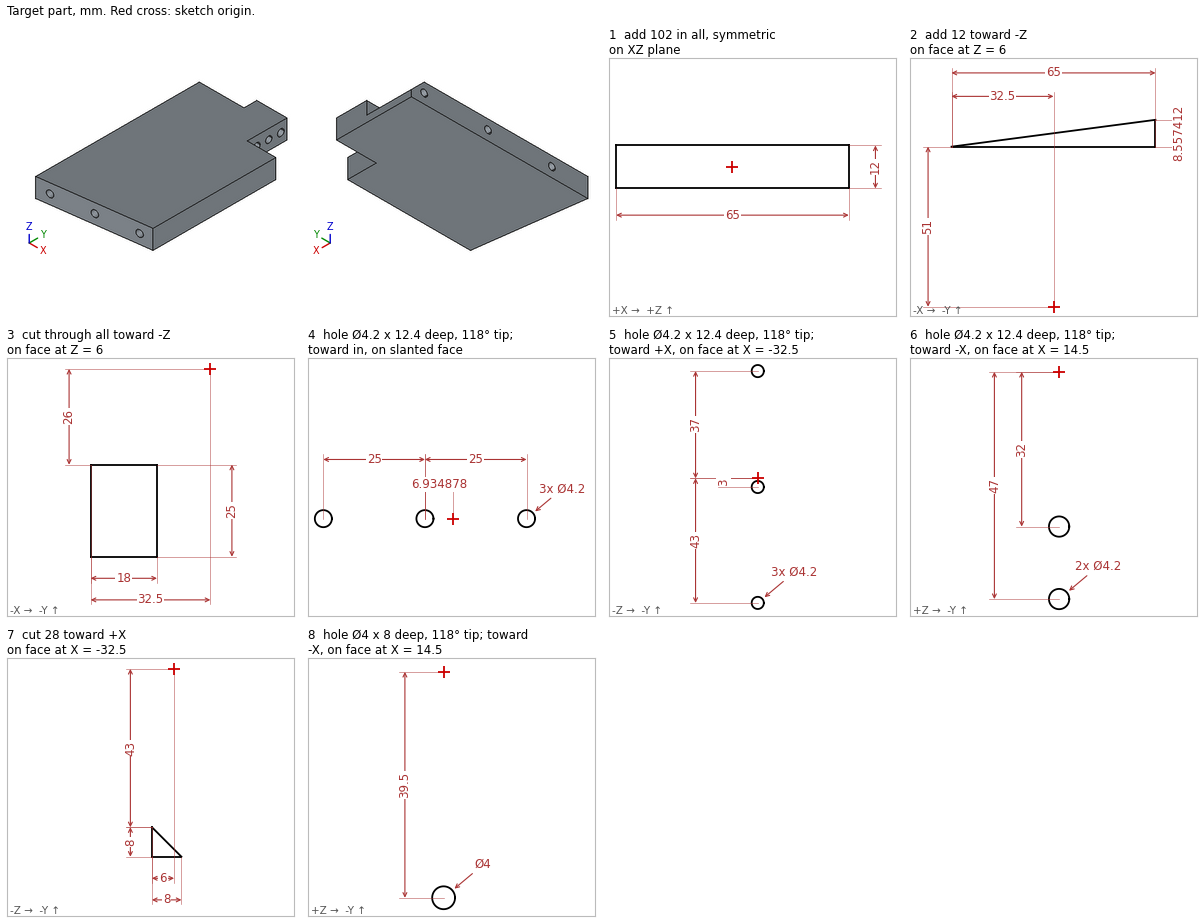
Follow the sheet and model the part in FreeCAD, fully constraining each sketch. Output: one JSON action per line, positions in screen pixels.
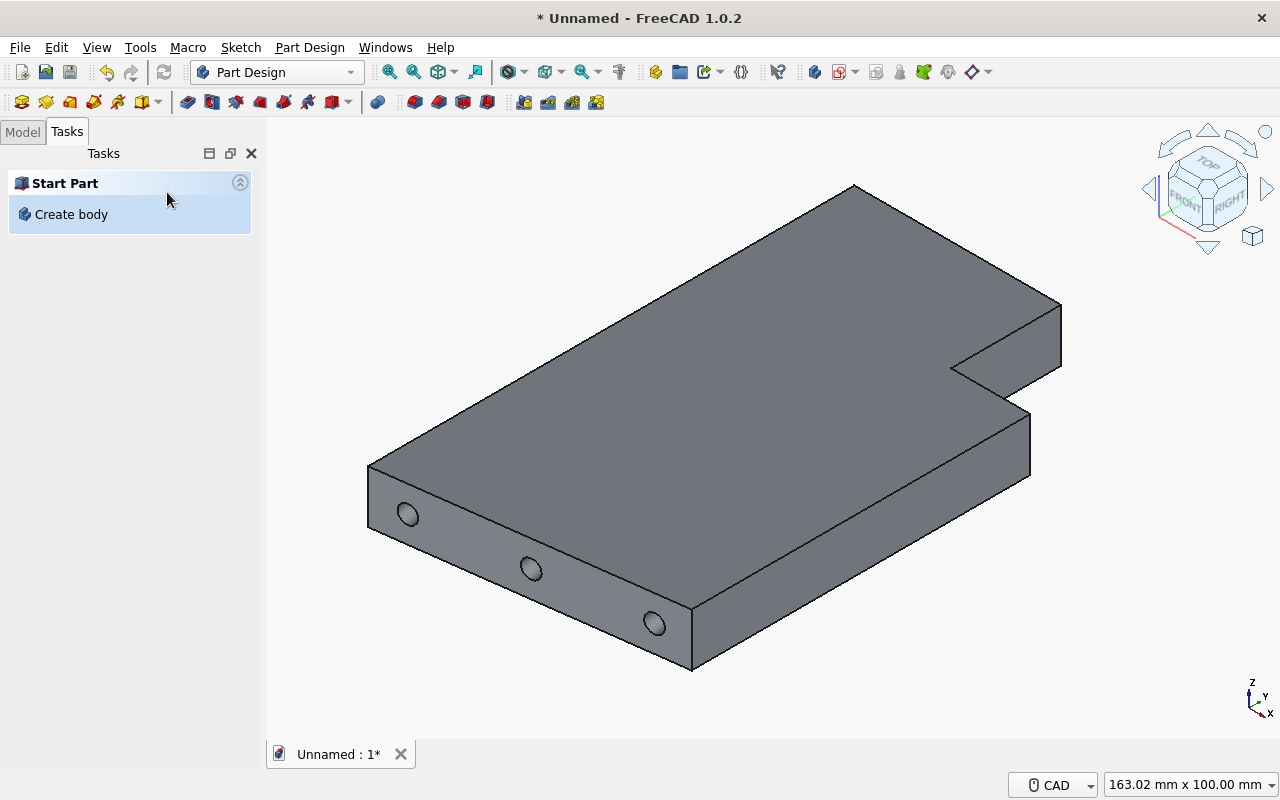
{"action": "left_click", "coordinate": [1022, 357]}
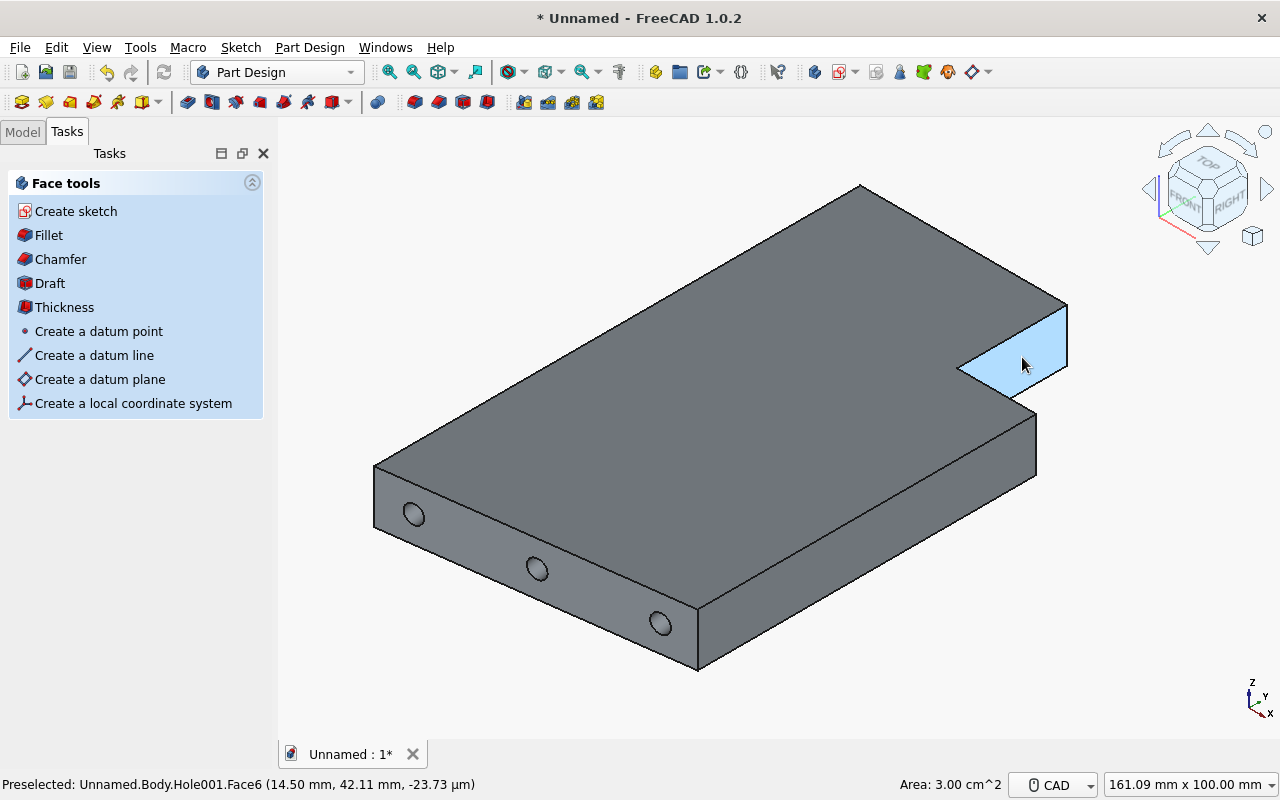
{"action": "left_click", "coordinate": [840, 72]}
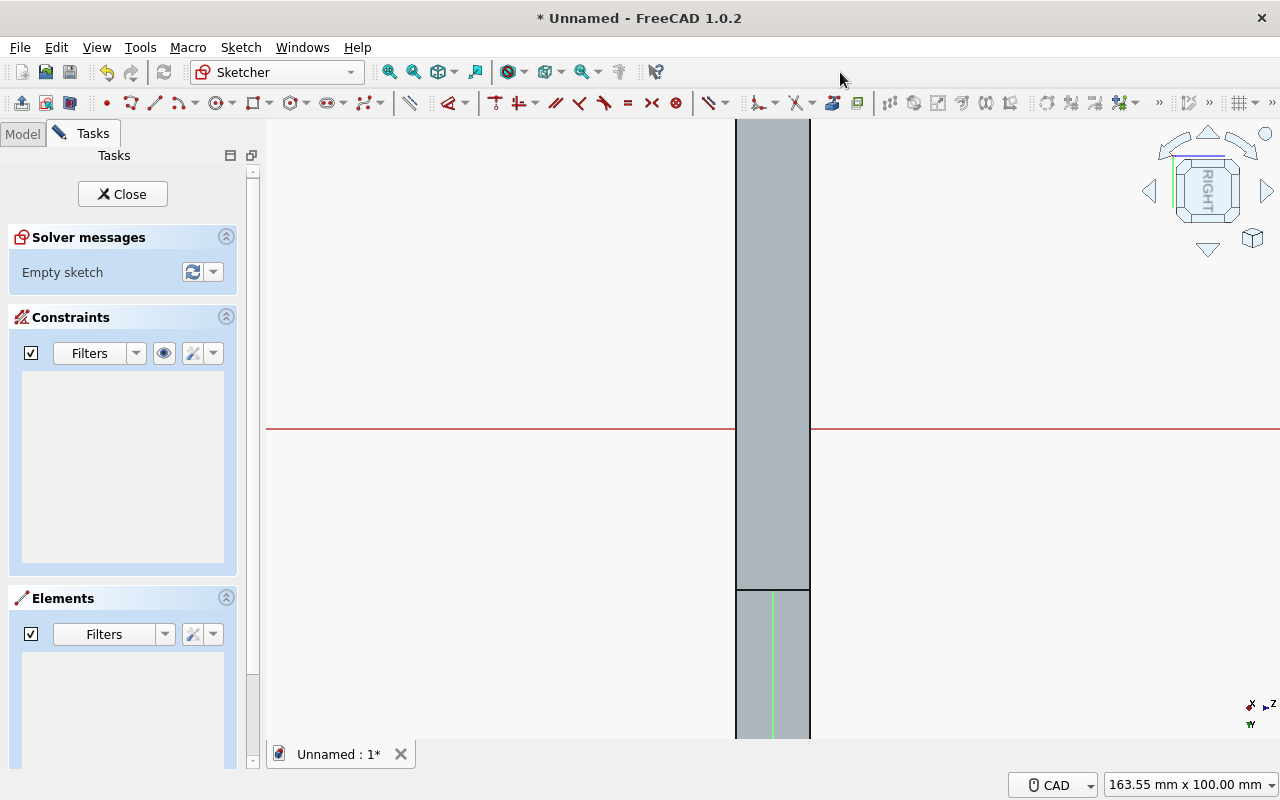
{"action": "scroll", "coordinate": [704, 429], "scroll_direction": "down", "scroll_amount": 5}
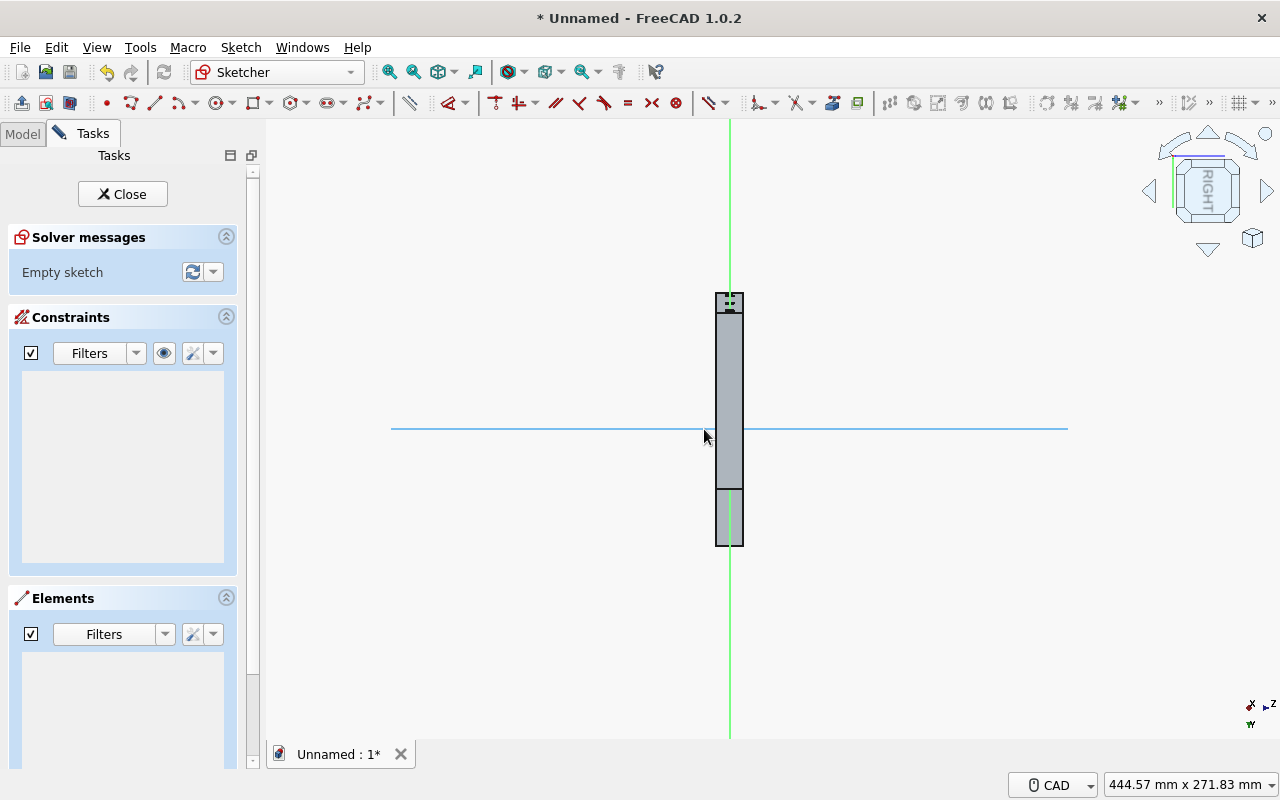
{"action": "scroll", "coordinate": [733, 531], "scroll_direction": "up", "scroll_amount": 11}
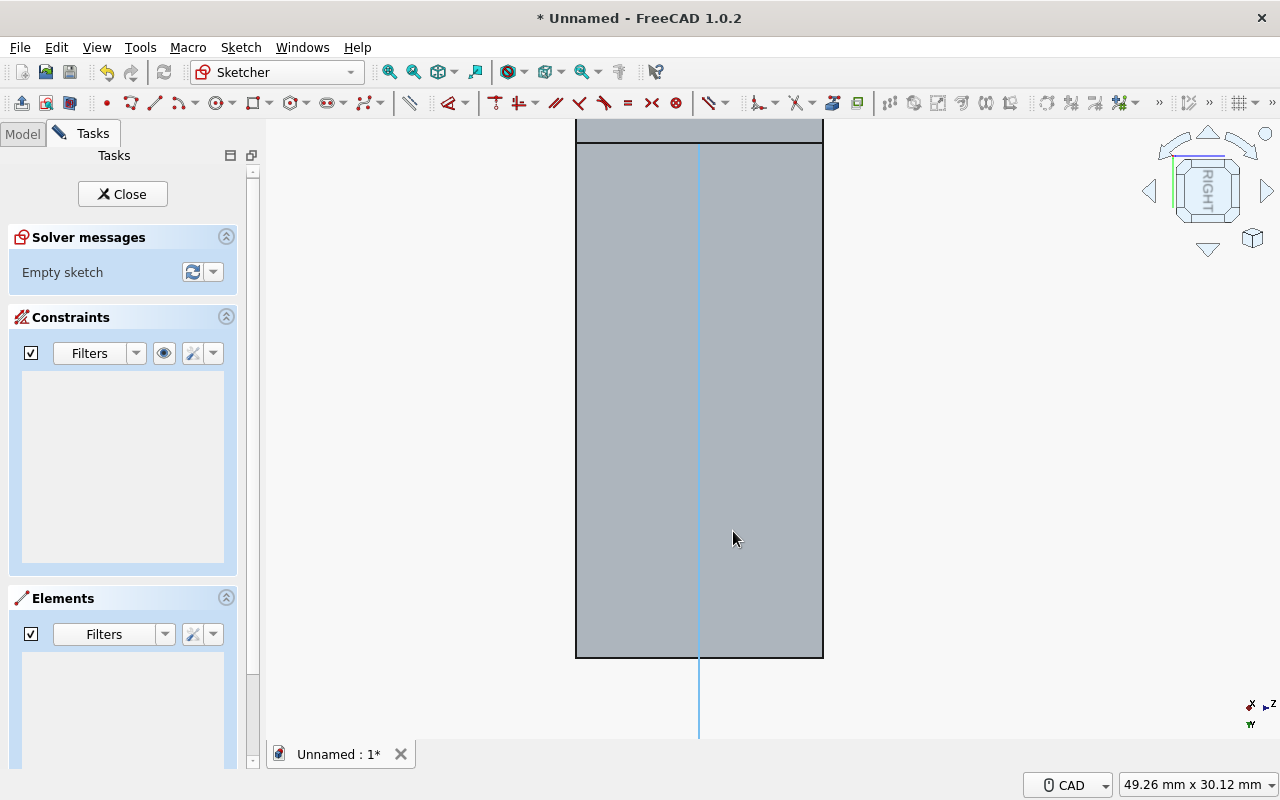
{"action": "key", "text": "g c"}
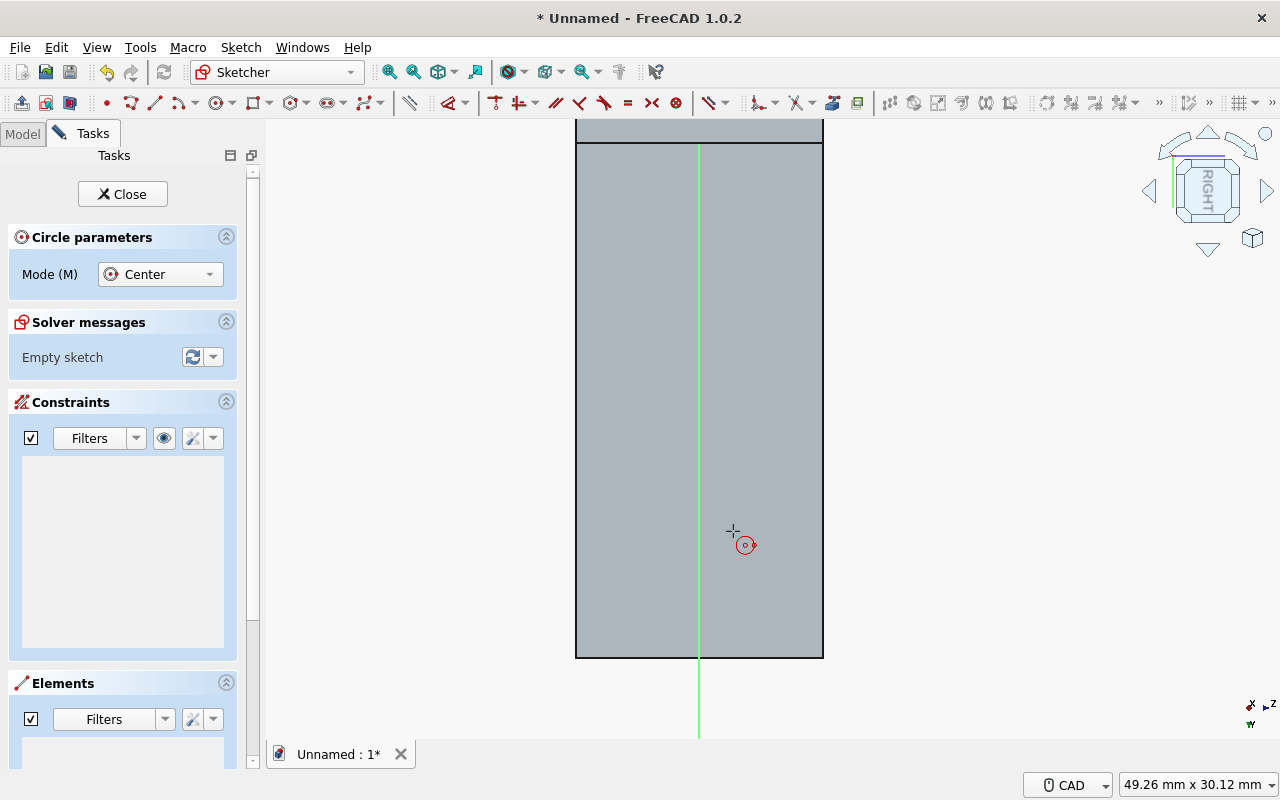
{"action": "left_click", "coordinate": [699, 575]}
{"action": "mouse_move", "coordinate": [730, 545]}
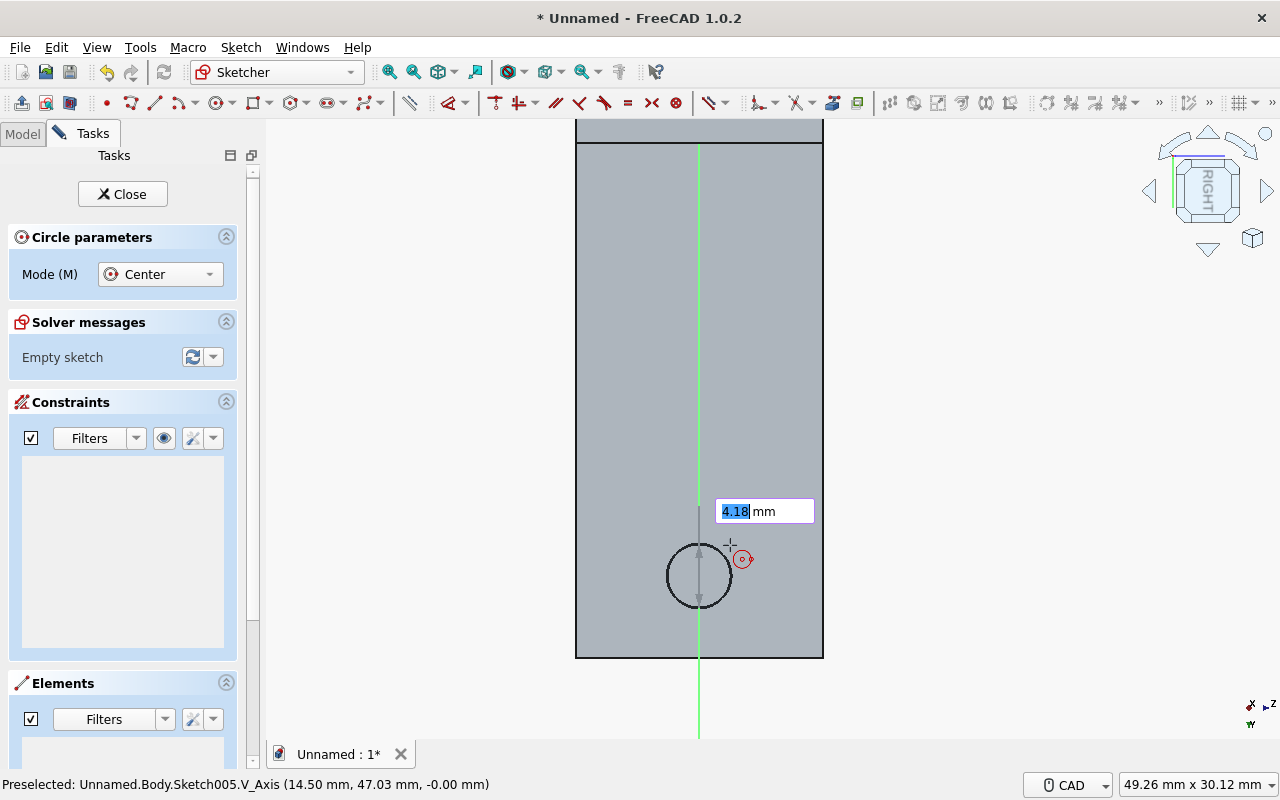
{"action": "type", "text": "4.2"}
{"action": "key", "text": "Return"}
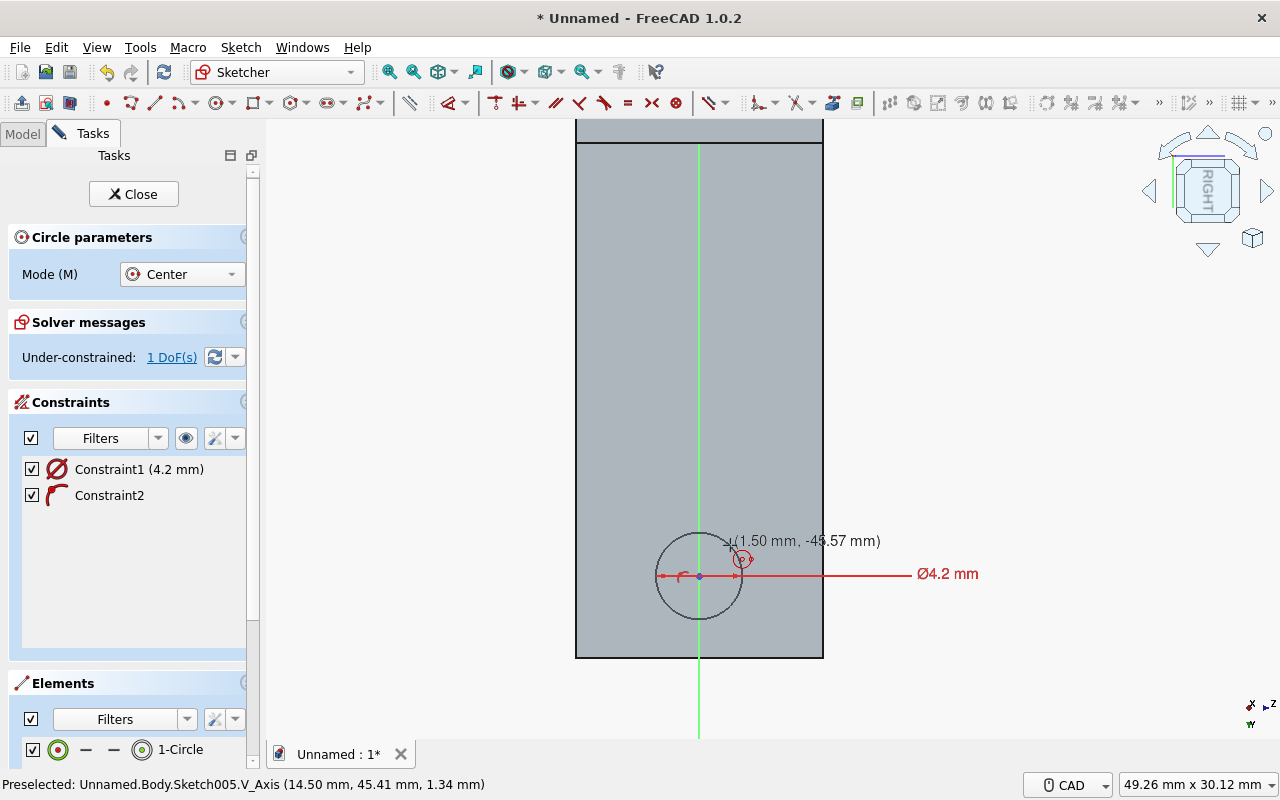
{"action": "left_click", "coordinate": [699, 267]}
{"action": "mouse_move", "coordinate": [730, 236]}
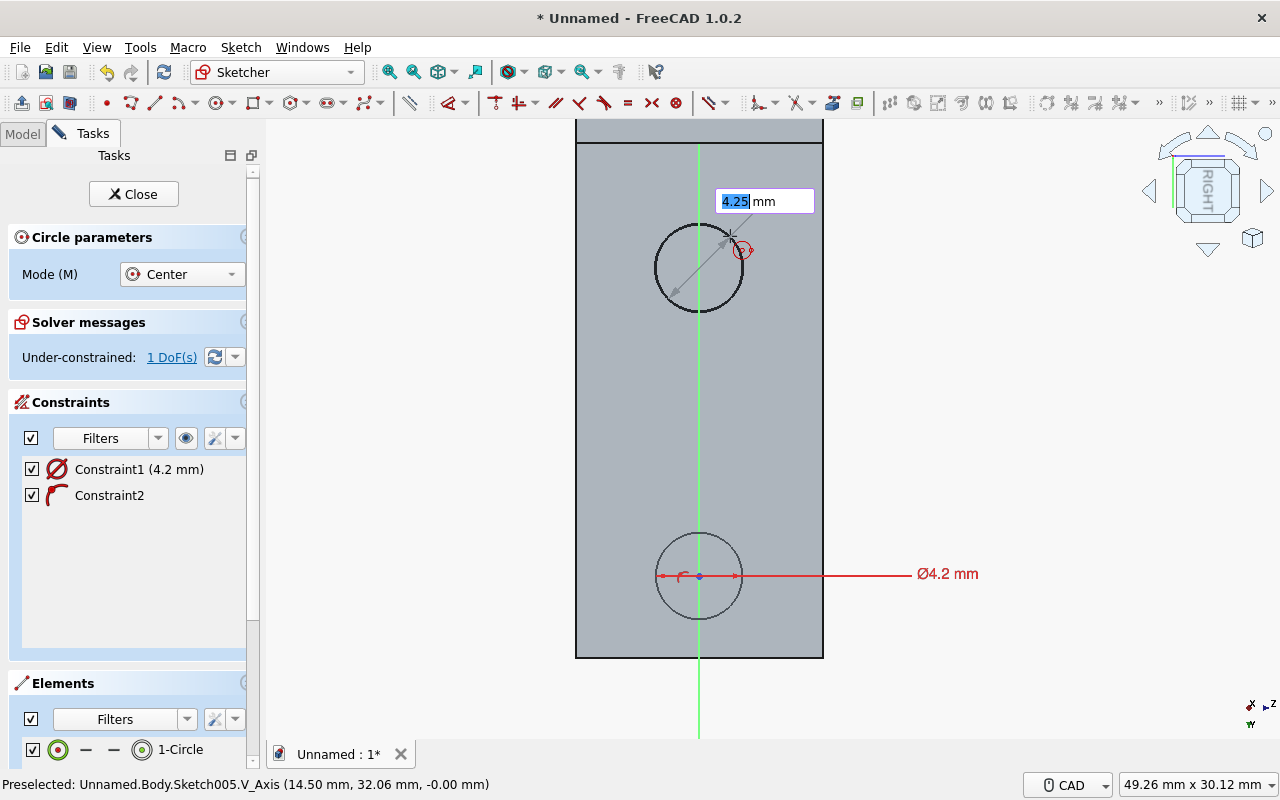
{"action": "type", "text": "4.2"}
{"action": "key", "text": "Return"}
{"action": "key", "text": "Escape"}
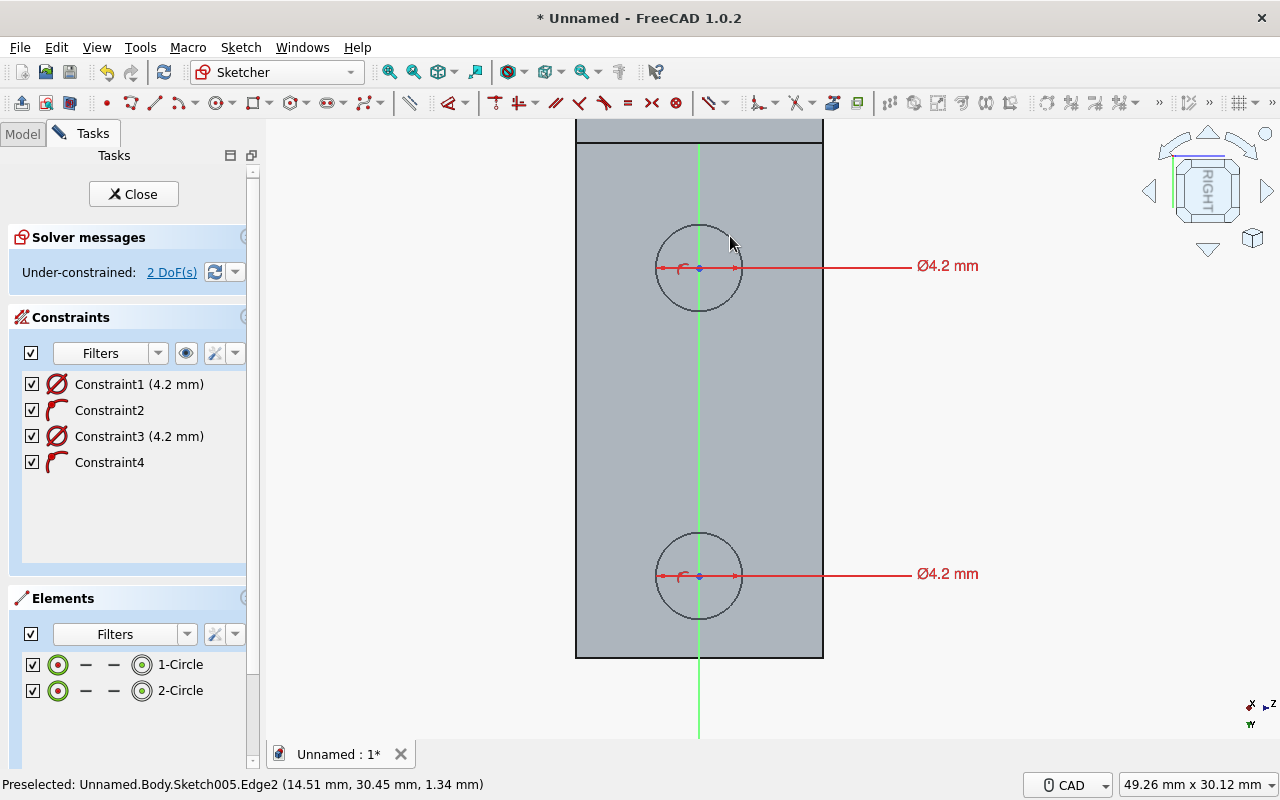
{"action": "key", "text": "d"}